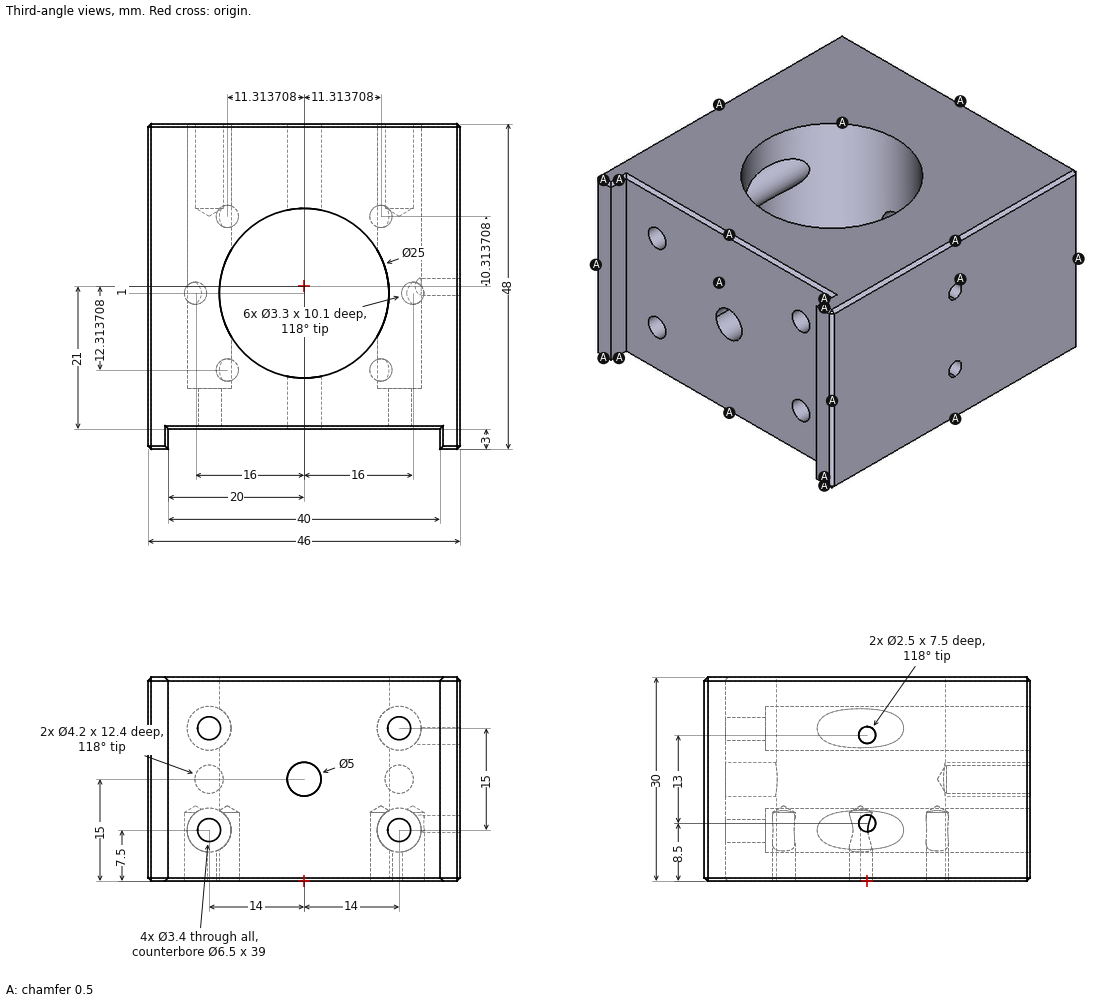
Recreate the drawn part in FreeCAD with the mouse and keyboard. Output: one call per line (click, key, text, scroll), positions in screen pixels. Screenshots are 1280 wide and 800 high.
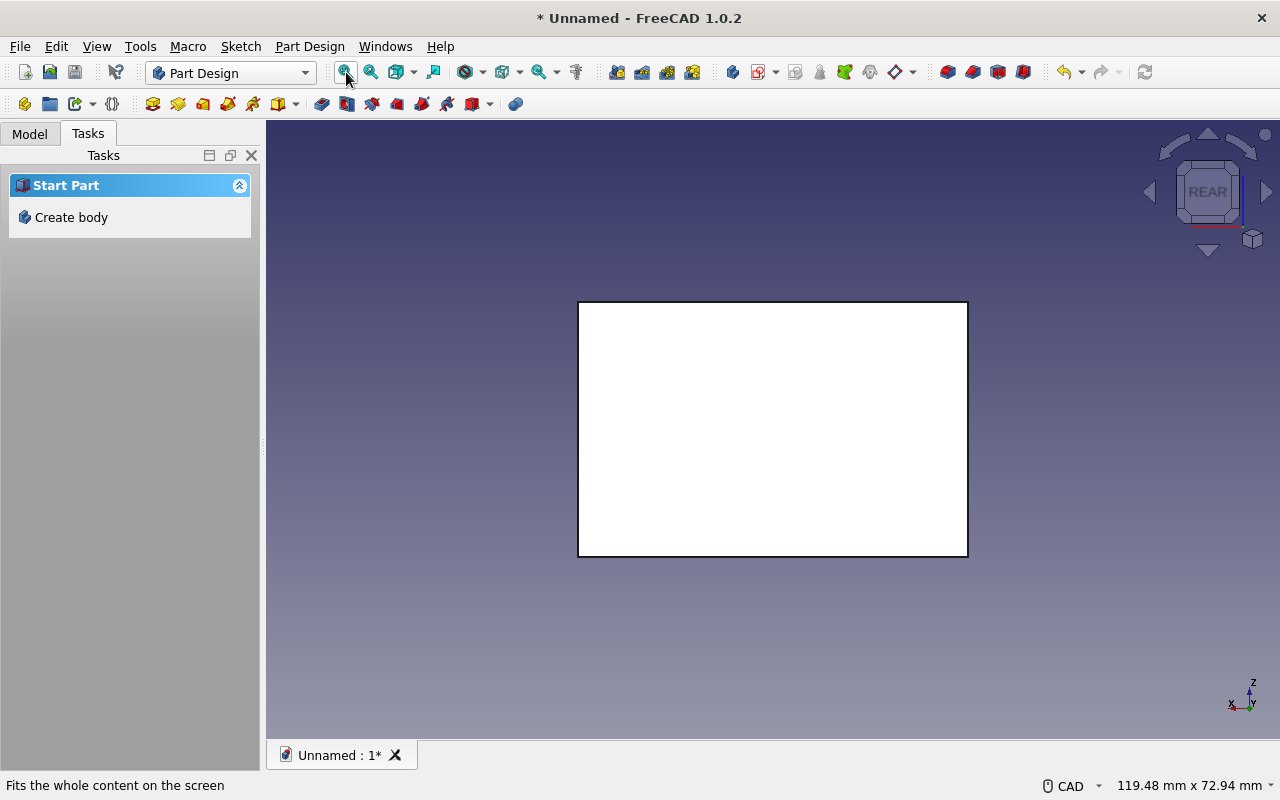
click(717, 429)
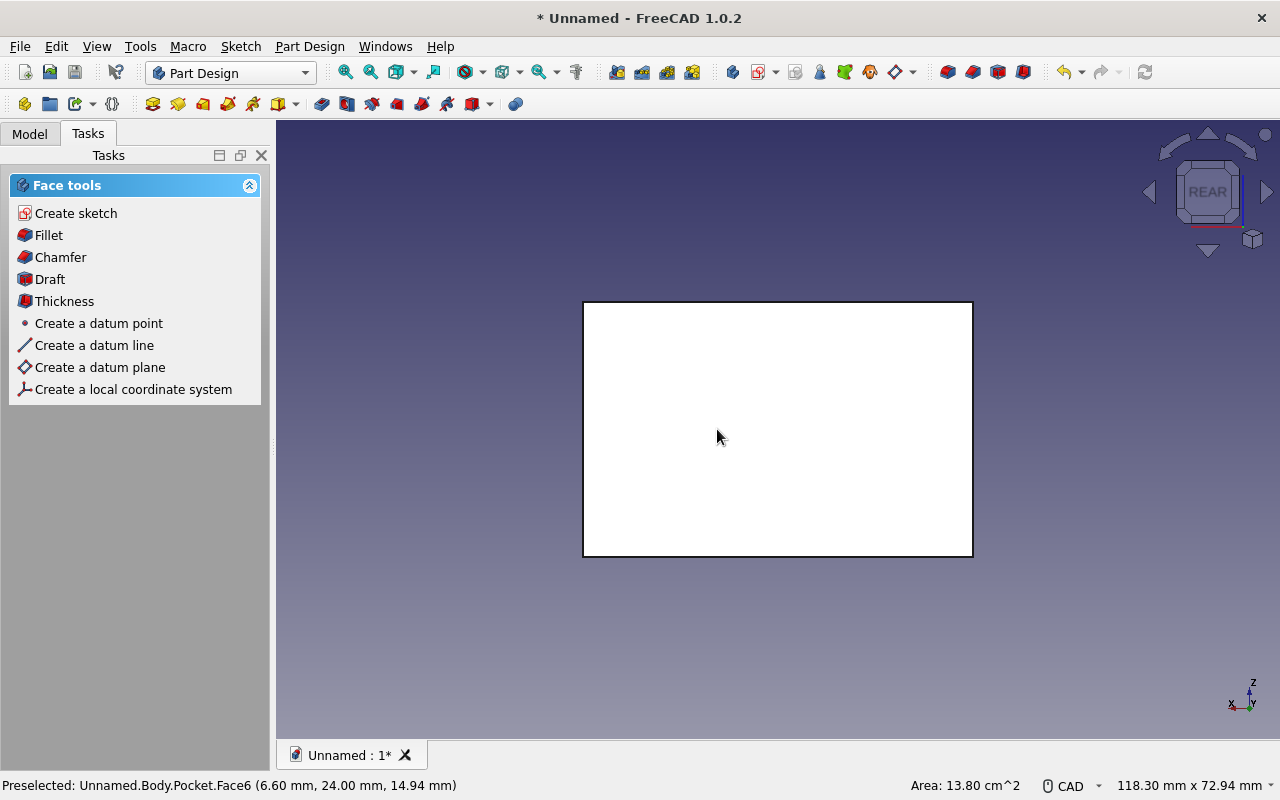
click(758, 72)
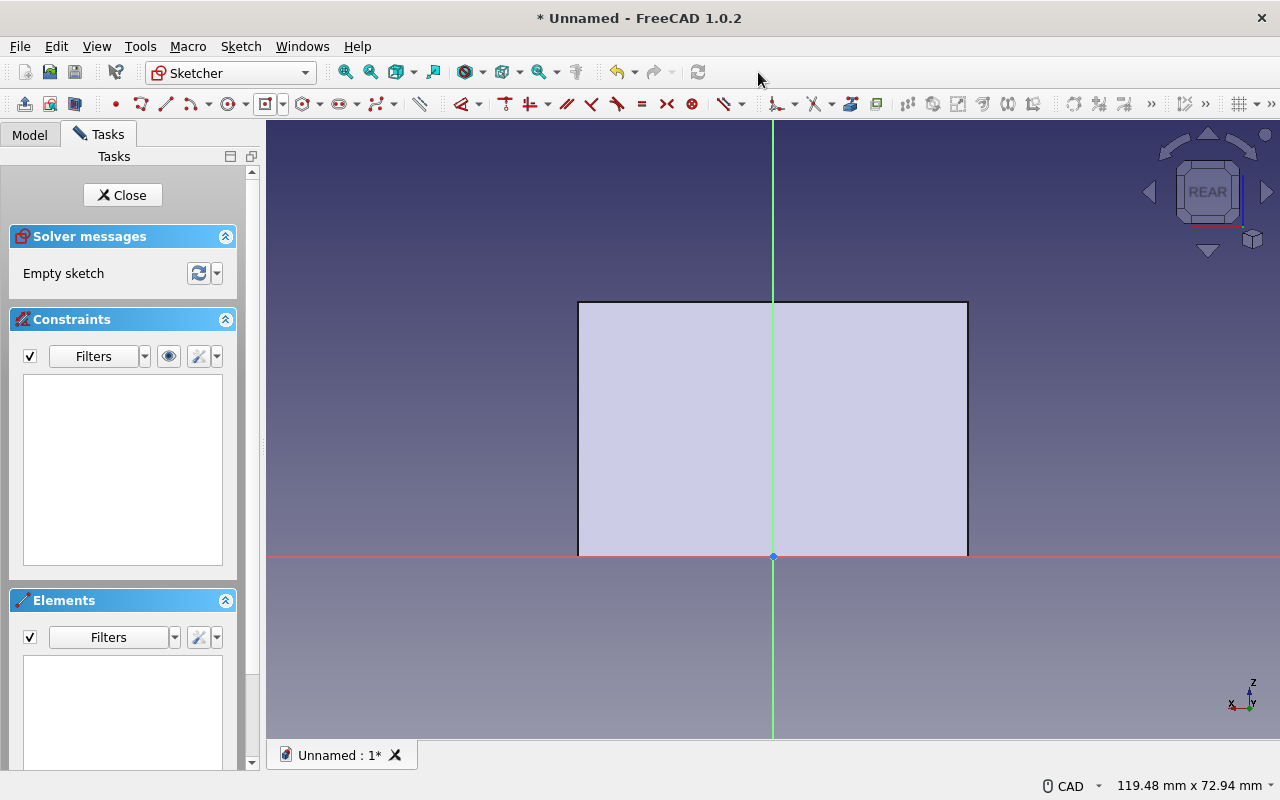
scroll(856, 484, up, 3)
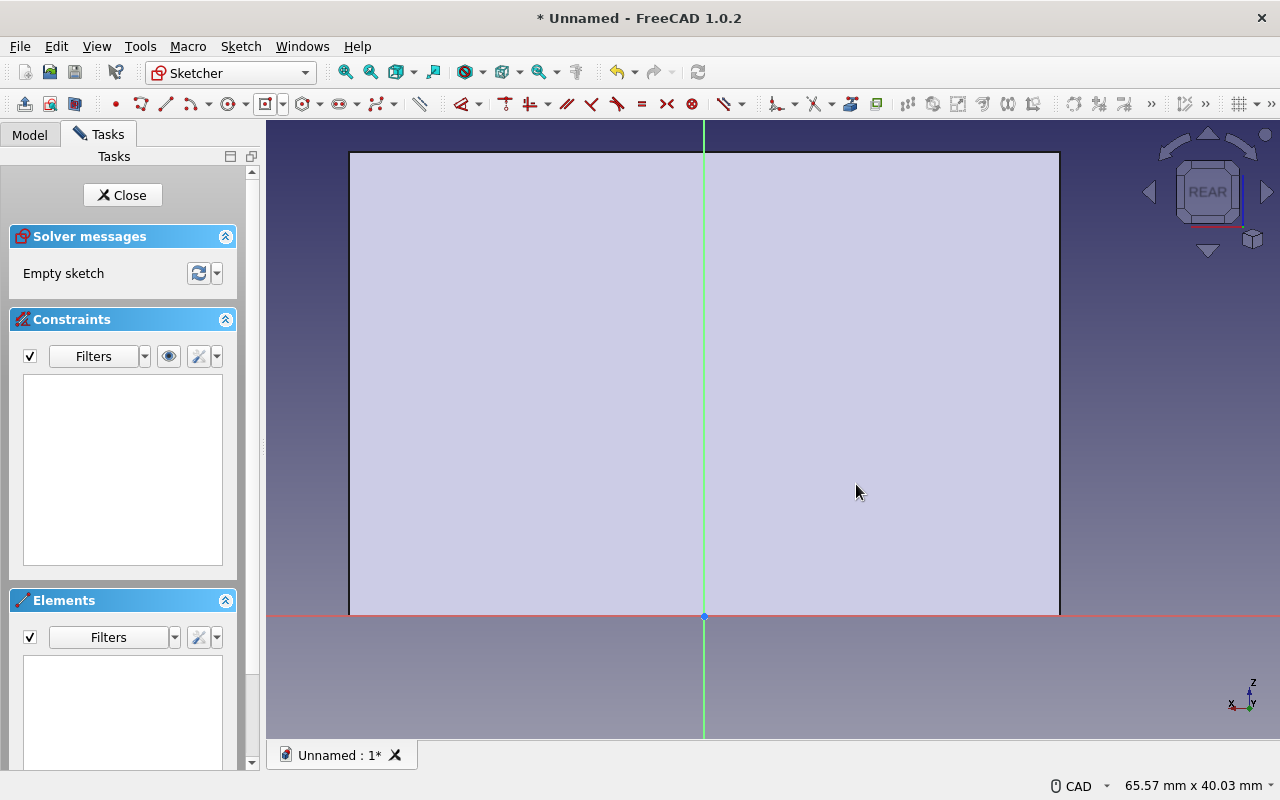
click(228, 104)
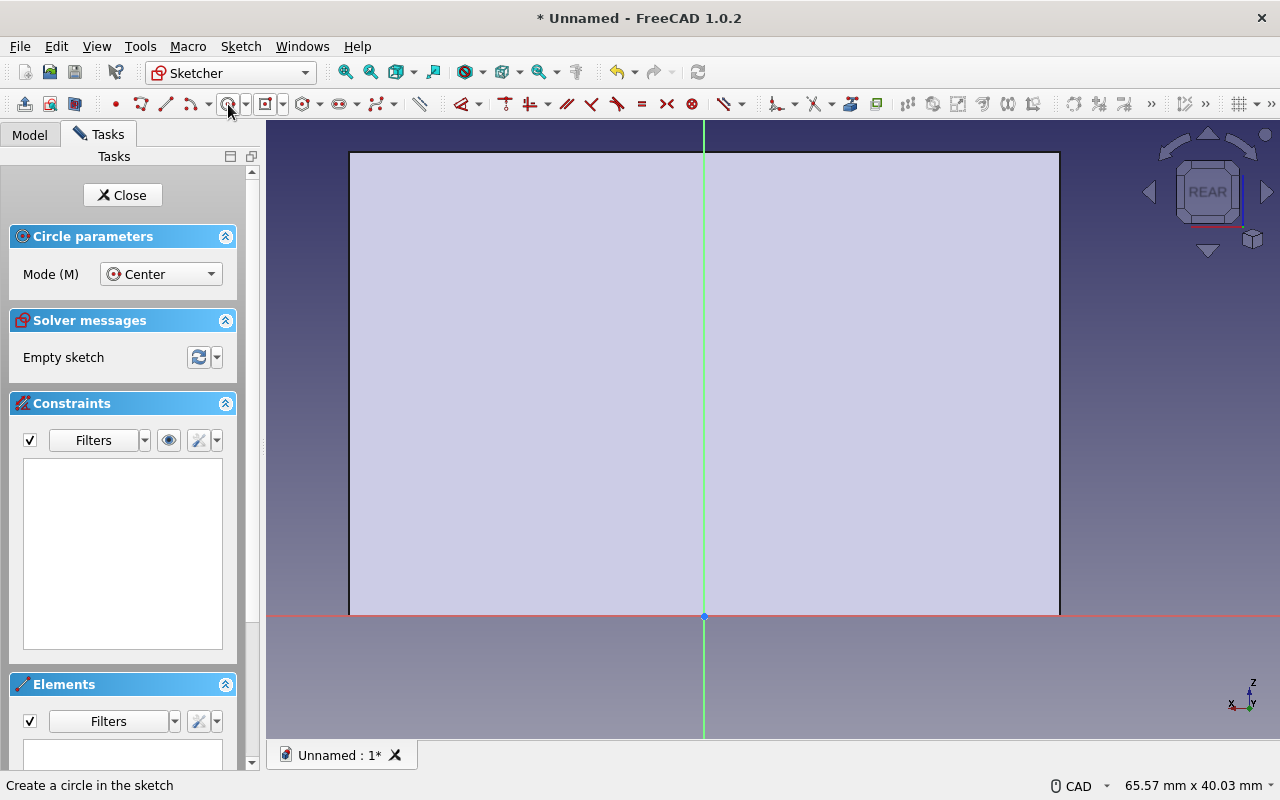
click(921, 500)
move(939, 482)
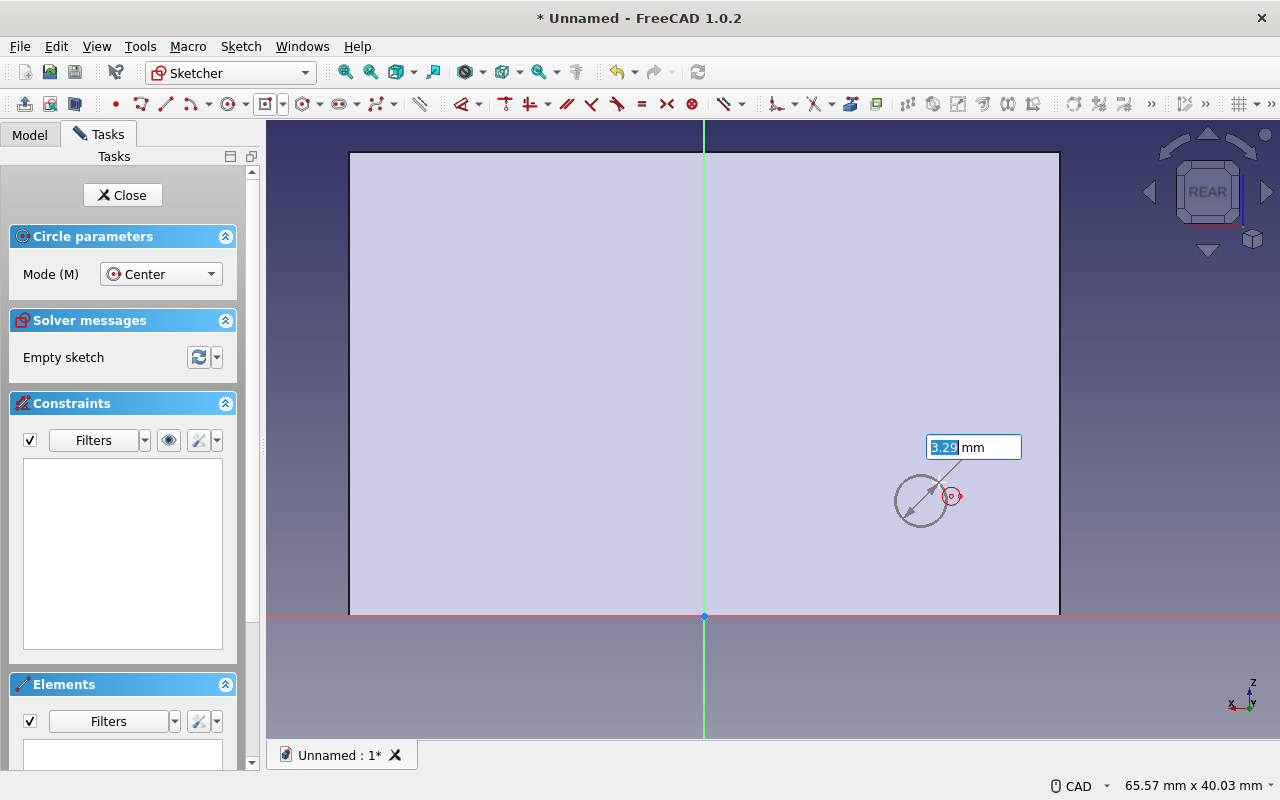
text(3.4)
key(Return)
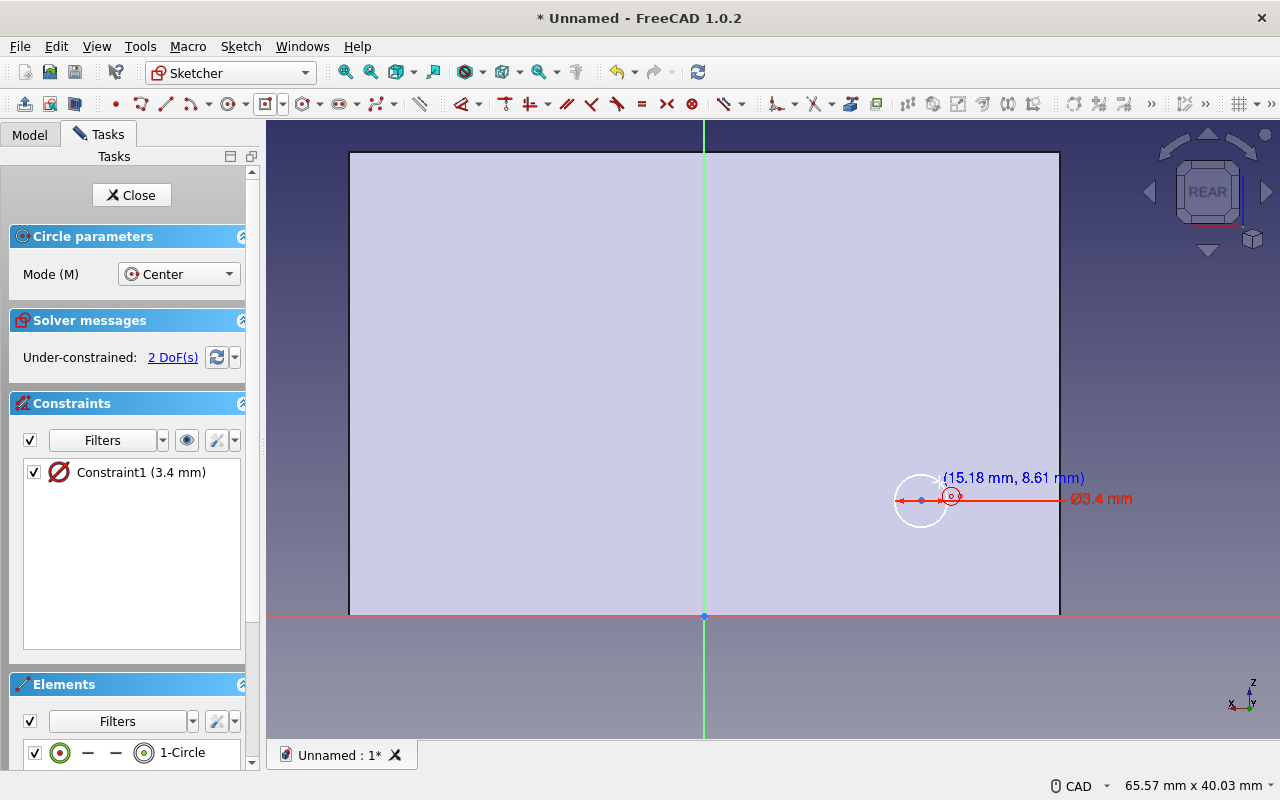
click(488, 500)
move(506, 482)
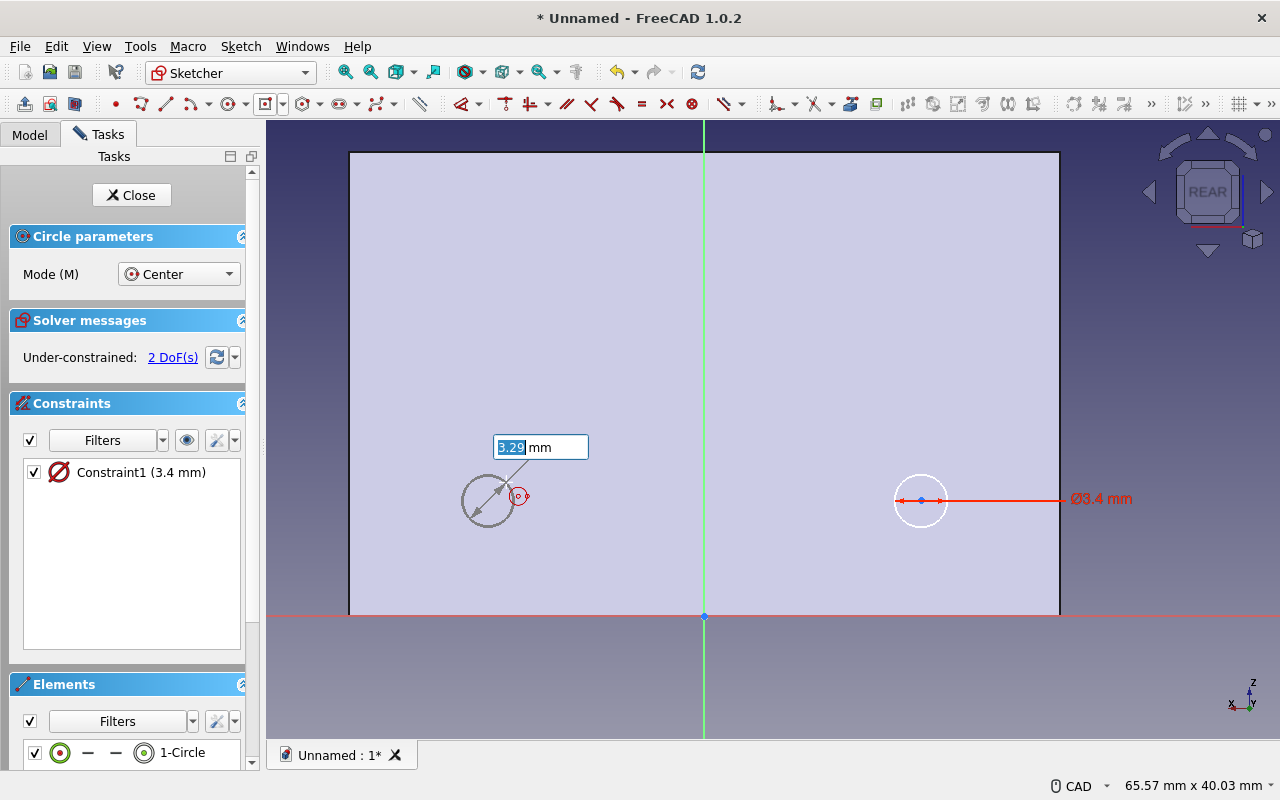
text(3.4)
key(Return)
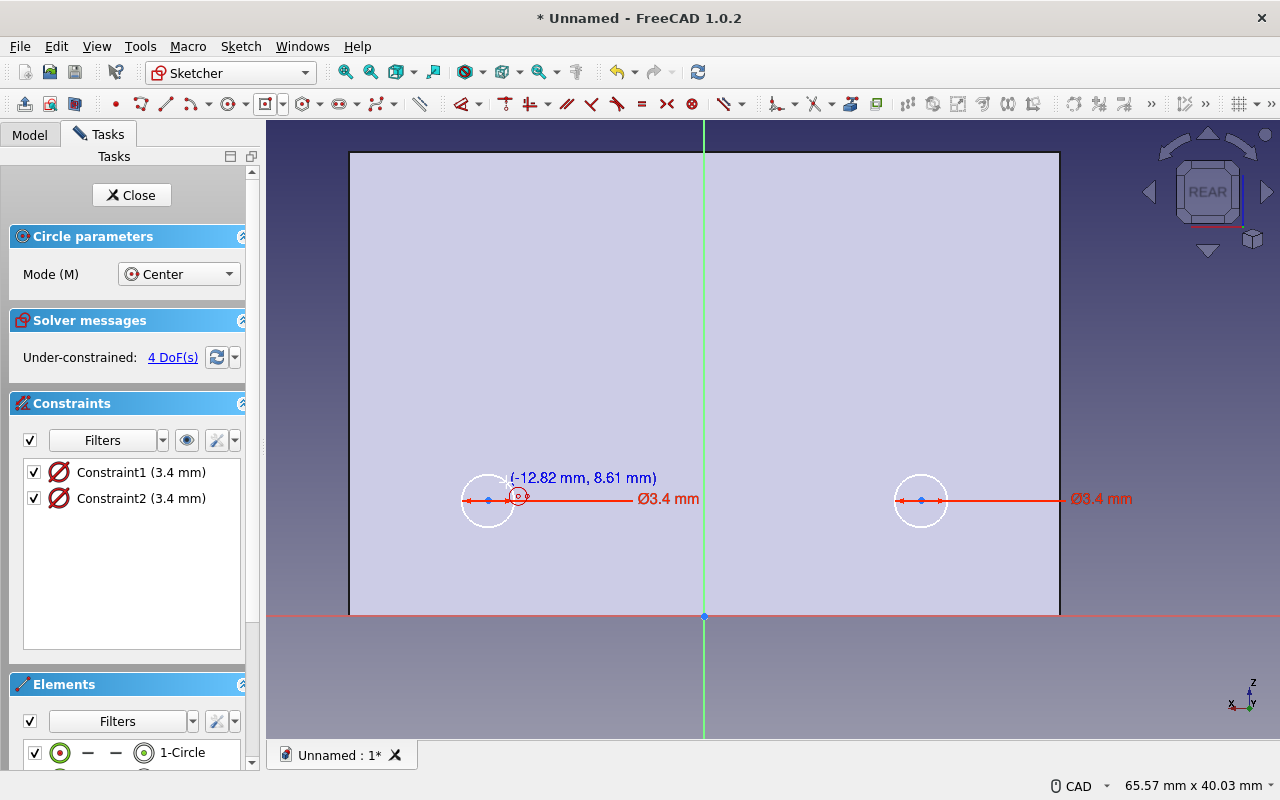
click(488, 268)
move(506, 250)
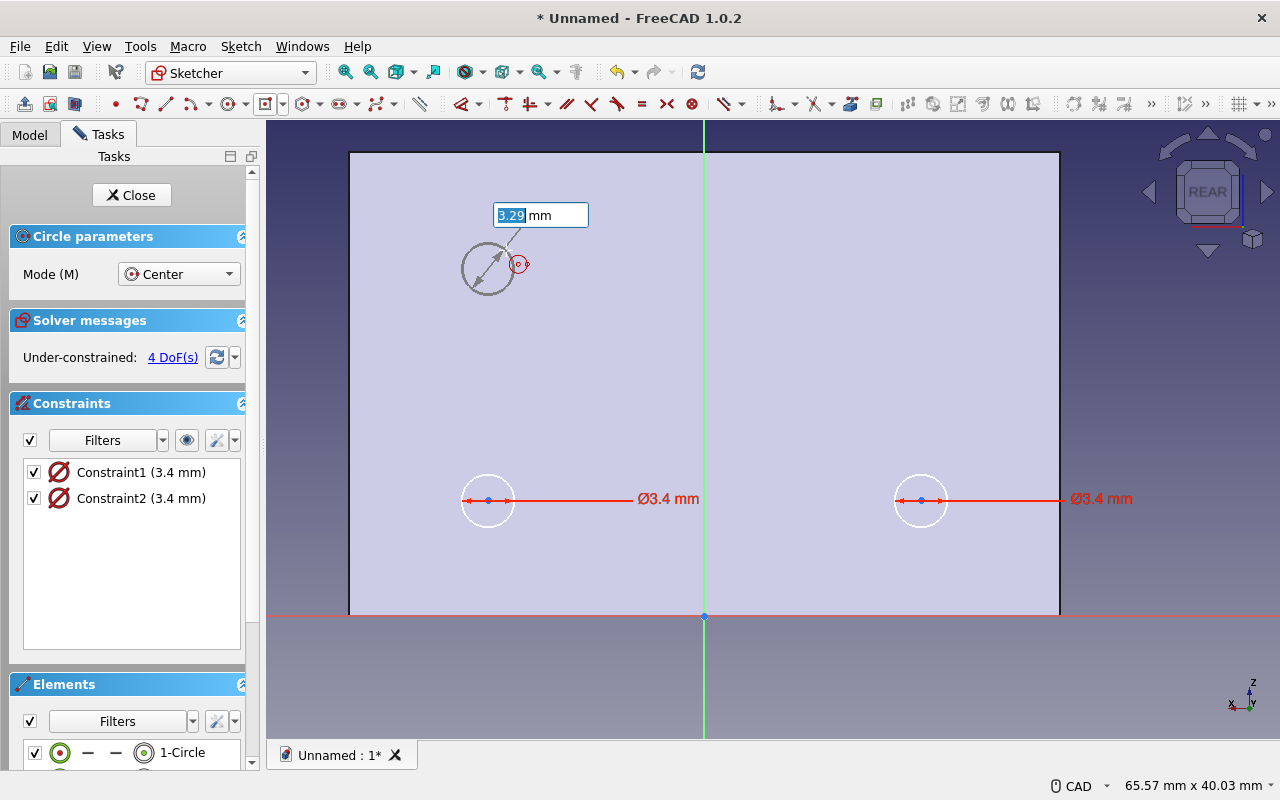
text(3.4)
key(Return)